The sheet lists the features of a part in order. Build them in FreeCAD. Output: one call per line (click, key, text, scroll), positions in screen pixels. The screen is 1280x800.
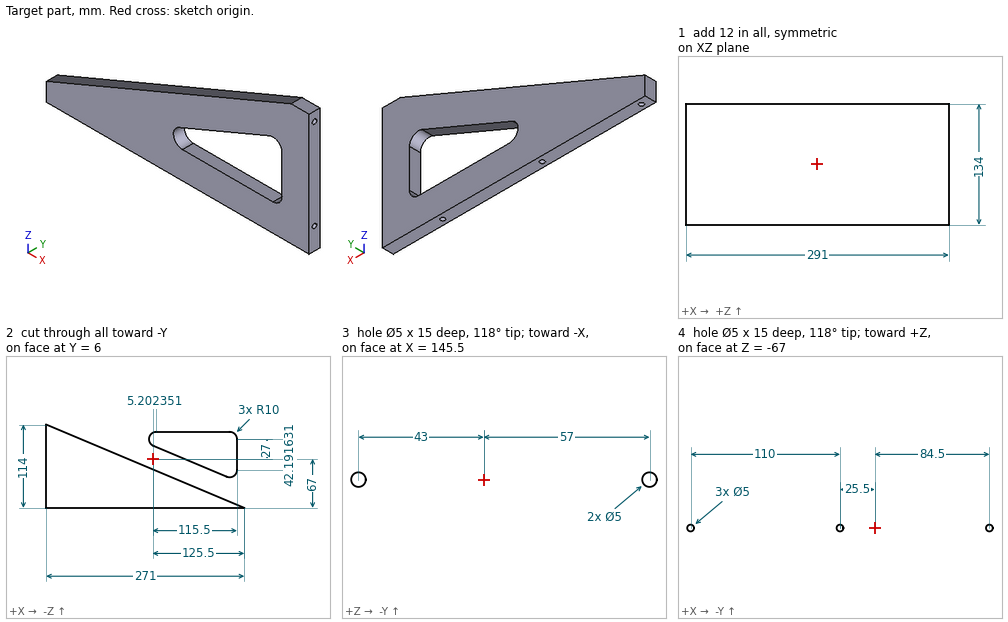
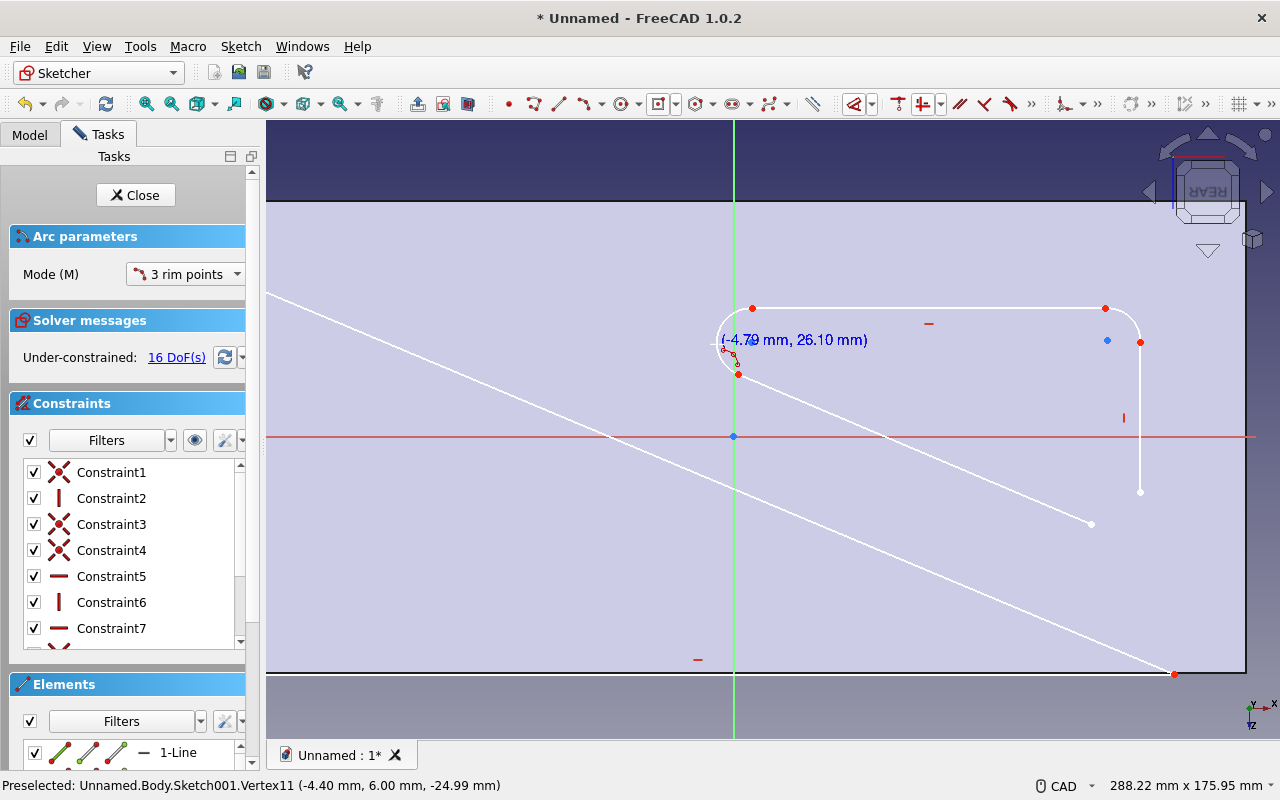
click(1091, 524)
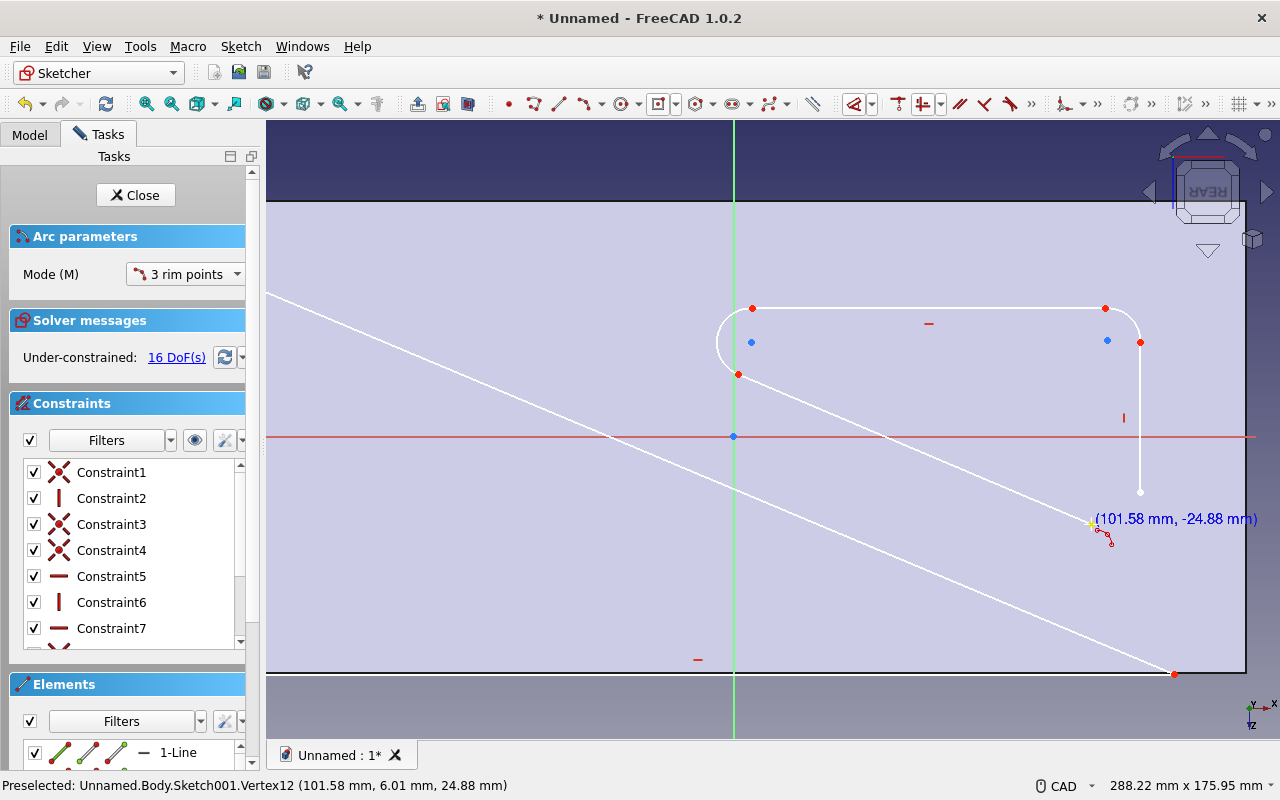
scroll(716, 343, down, 2)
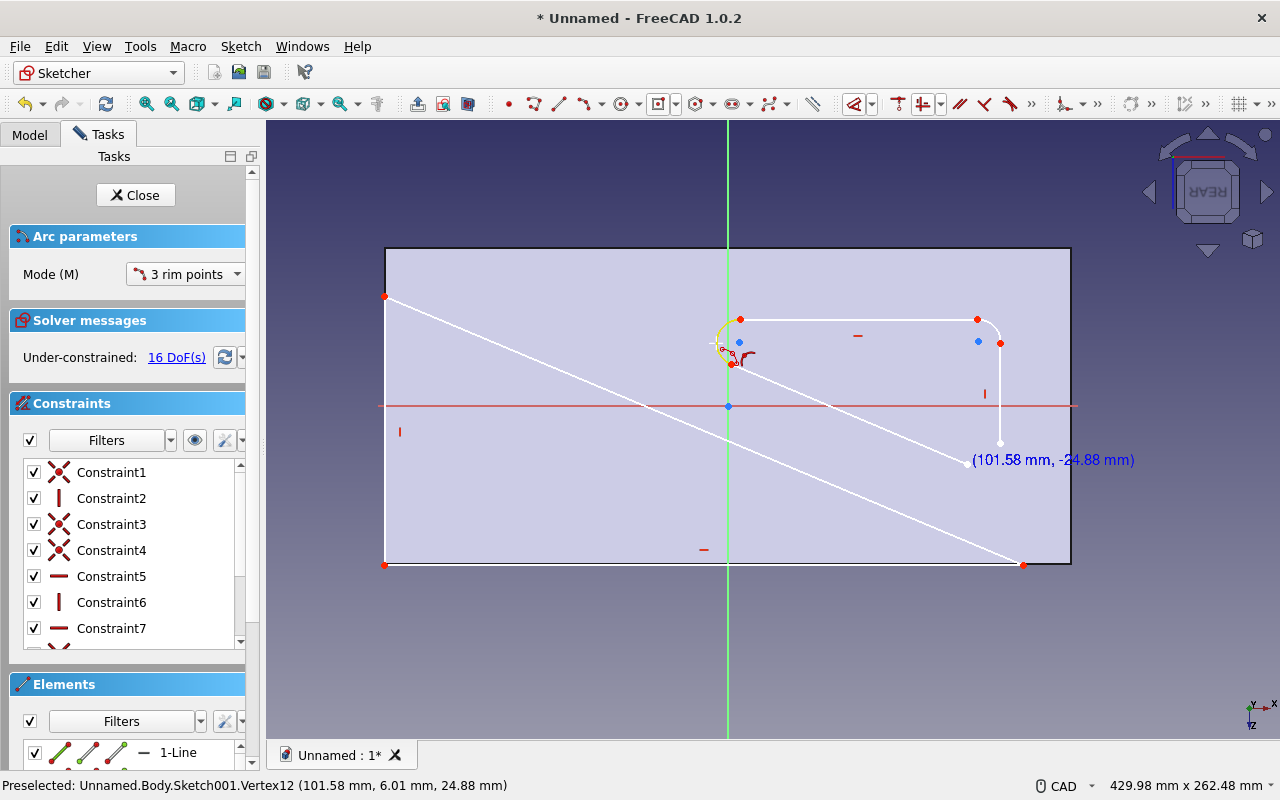
click(1000, 443)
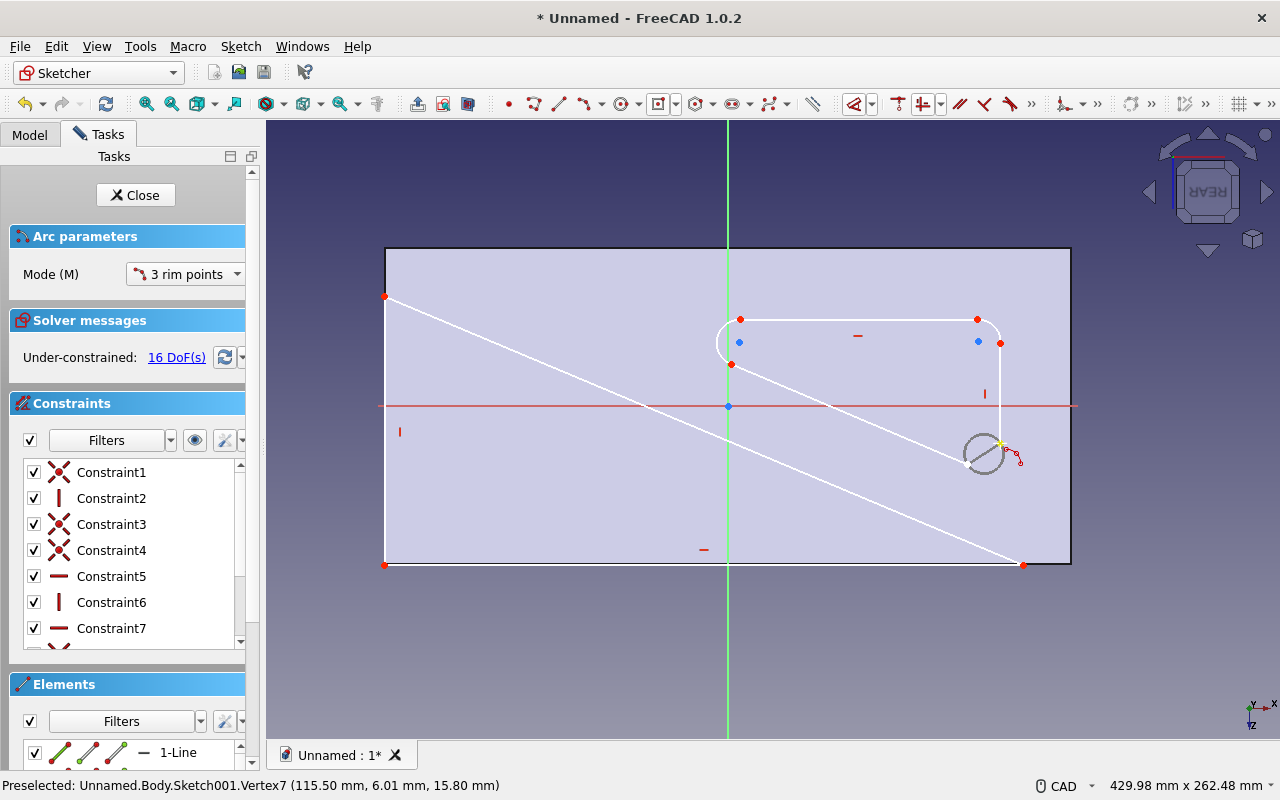
scroll(990, 461, up, 3)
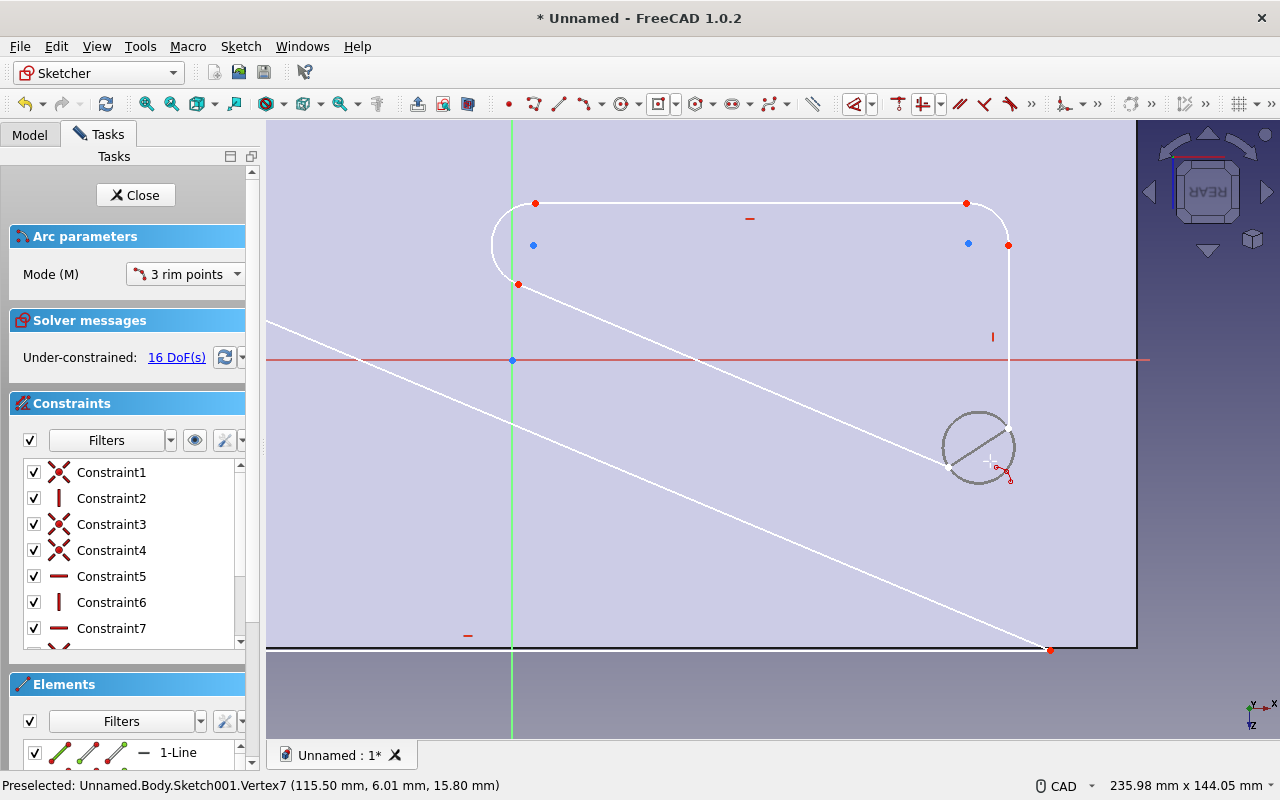
click(989, 461)
key(Escape)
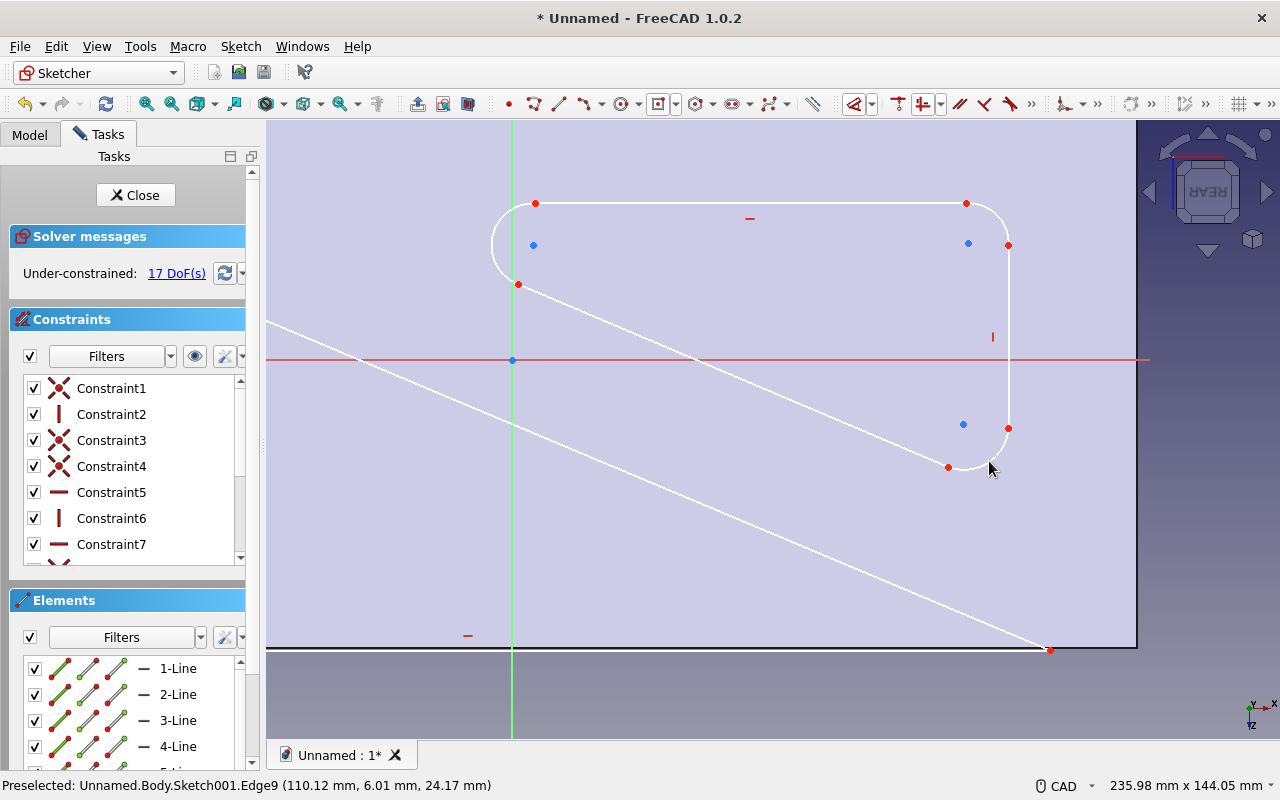
click(1009, 373)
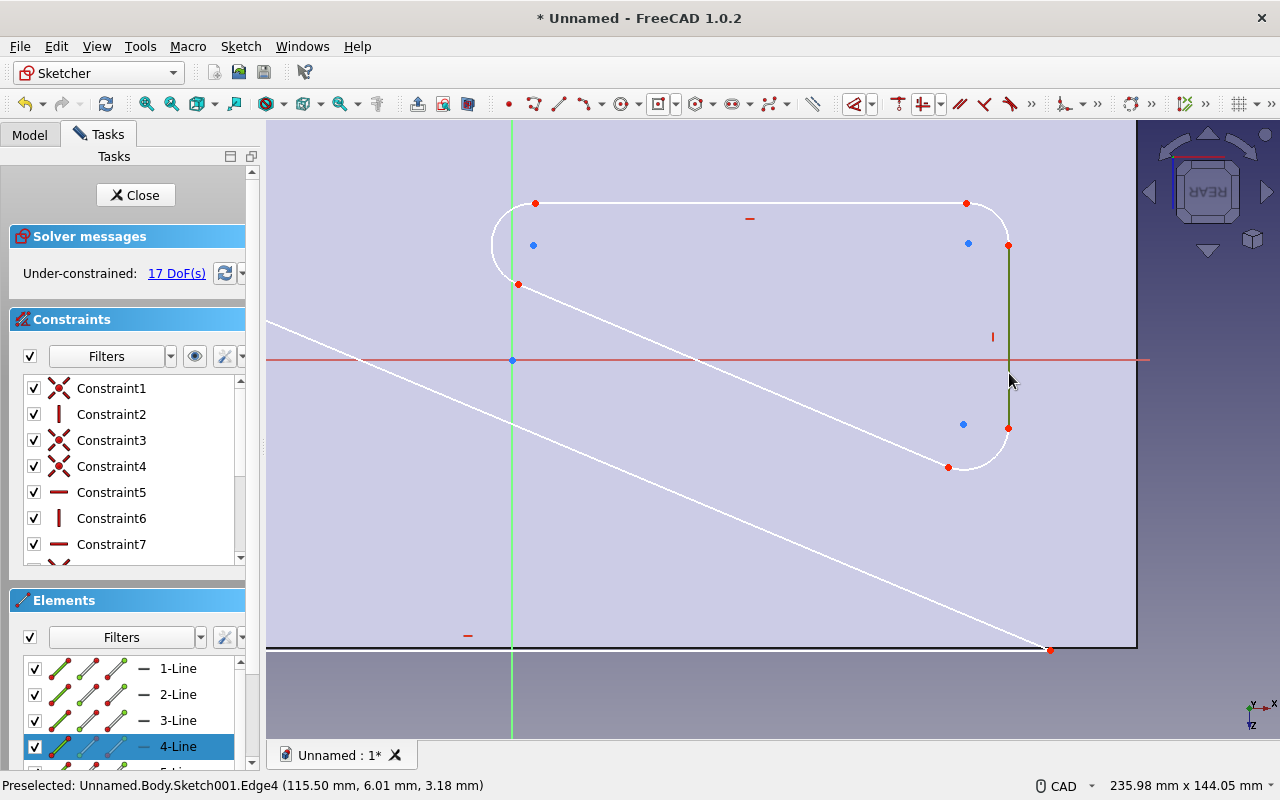
click(1005, 226)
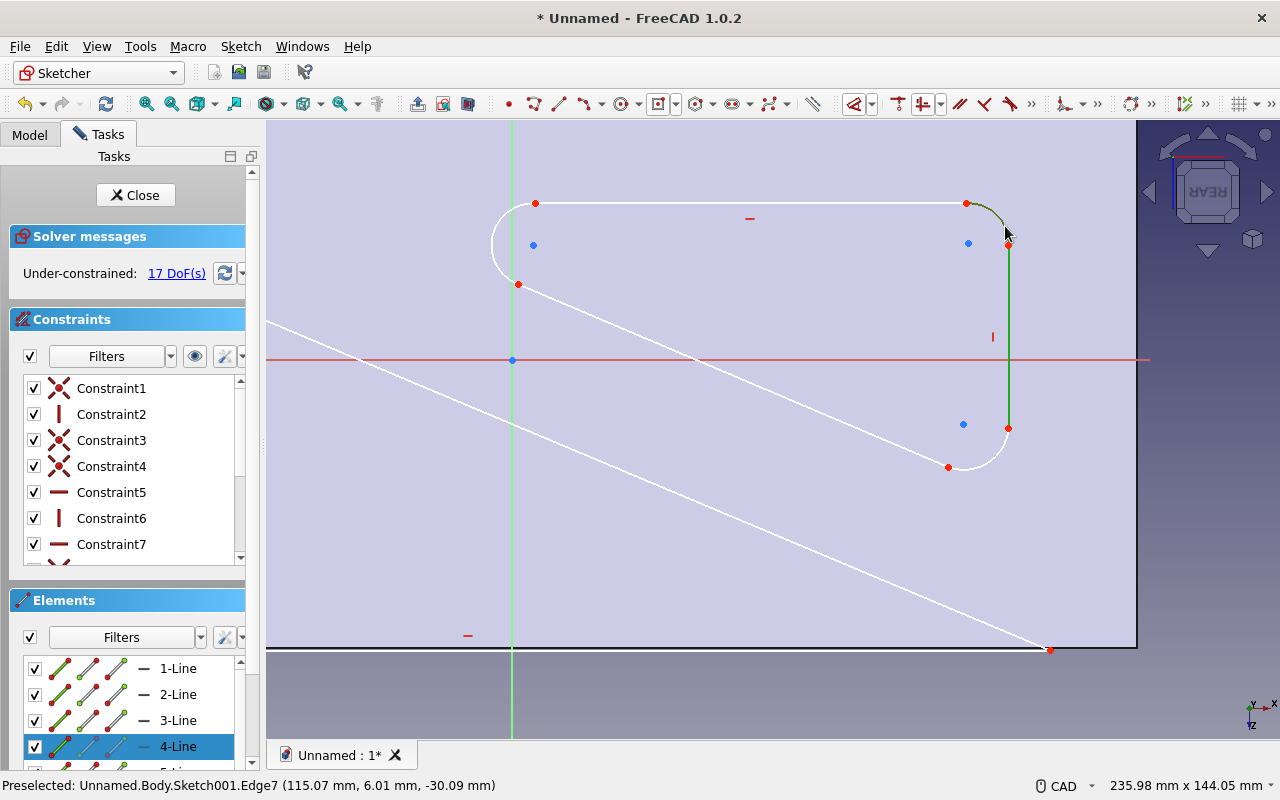
click(1010, 104)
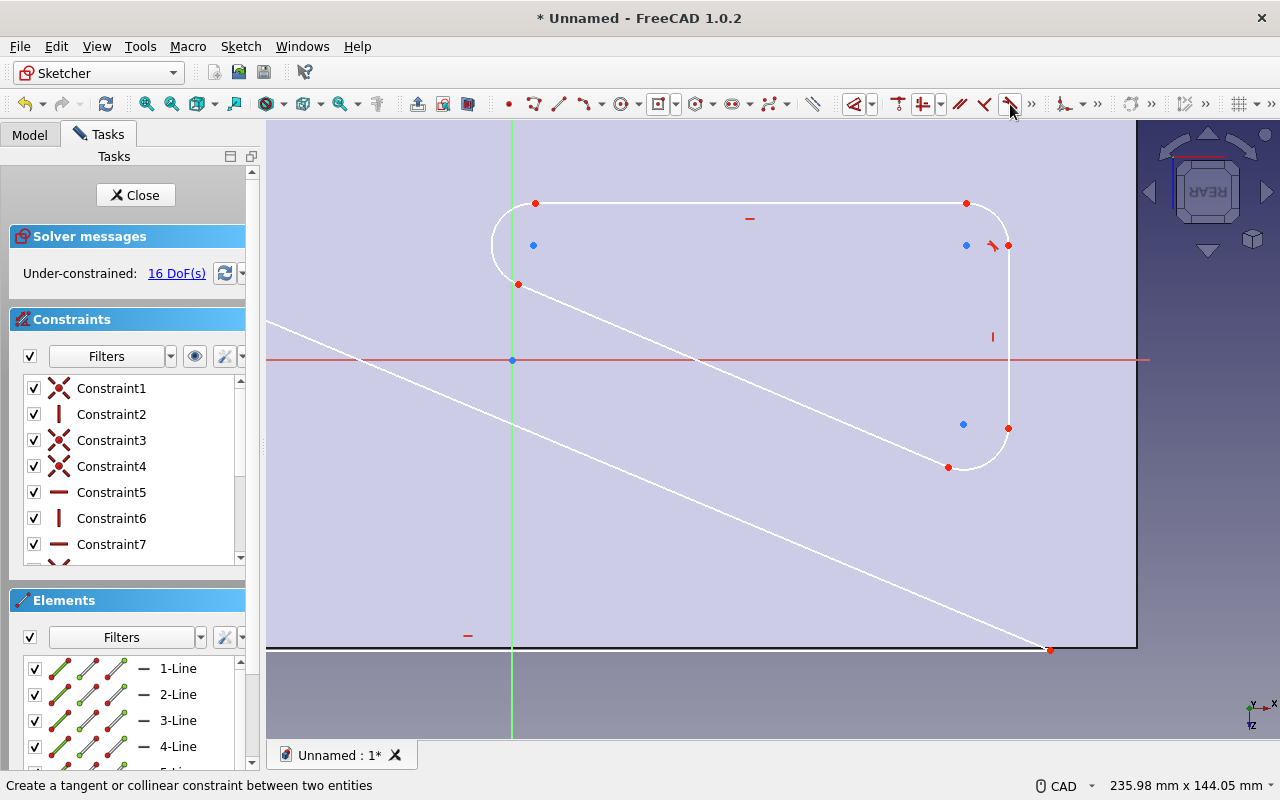
click(1009, 373)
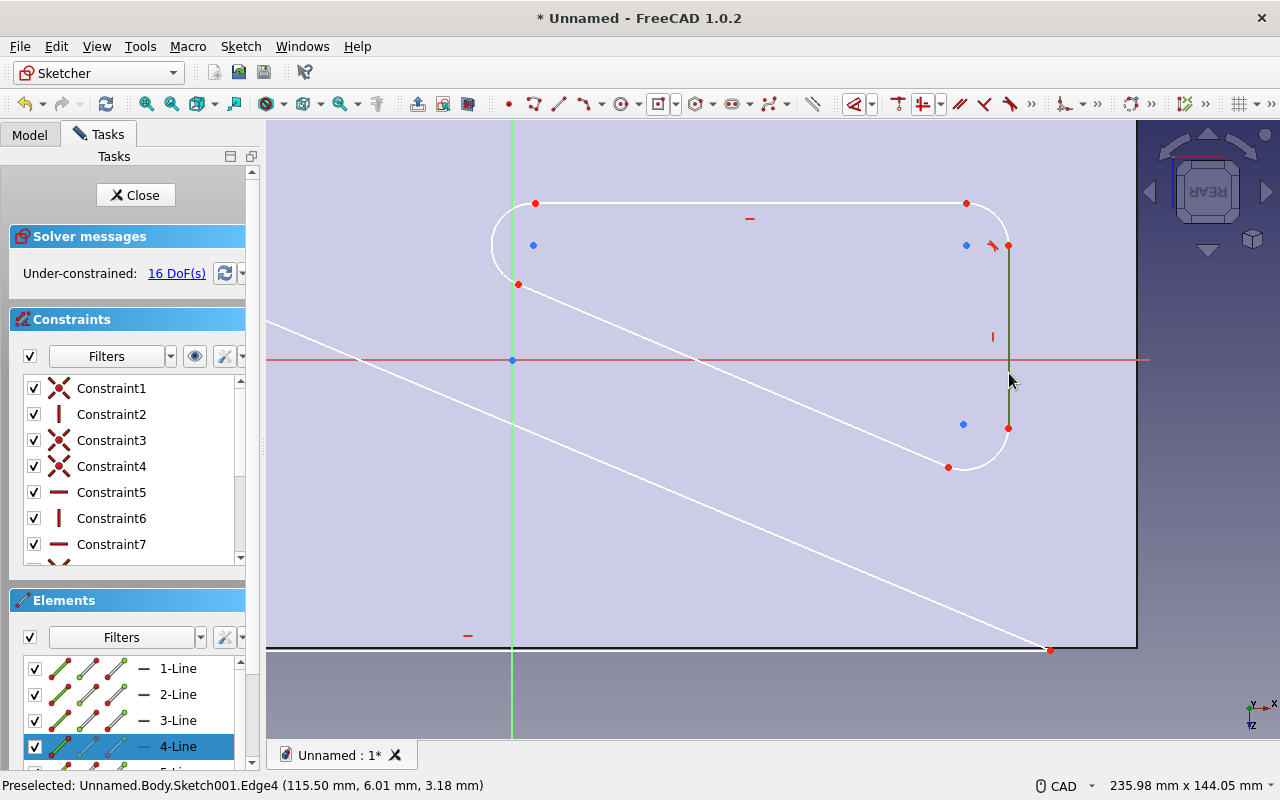
click(973, 469)